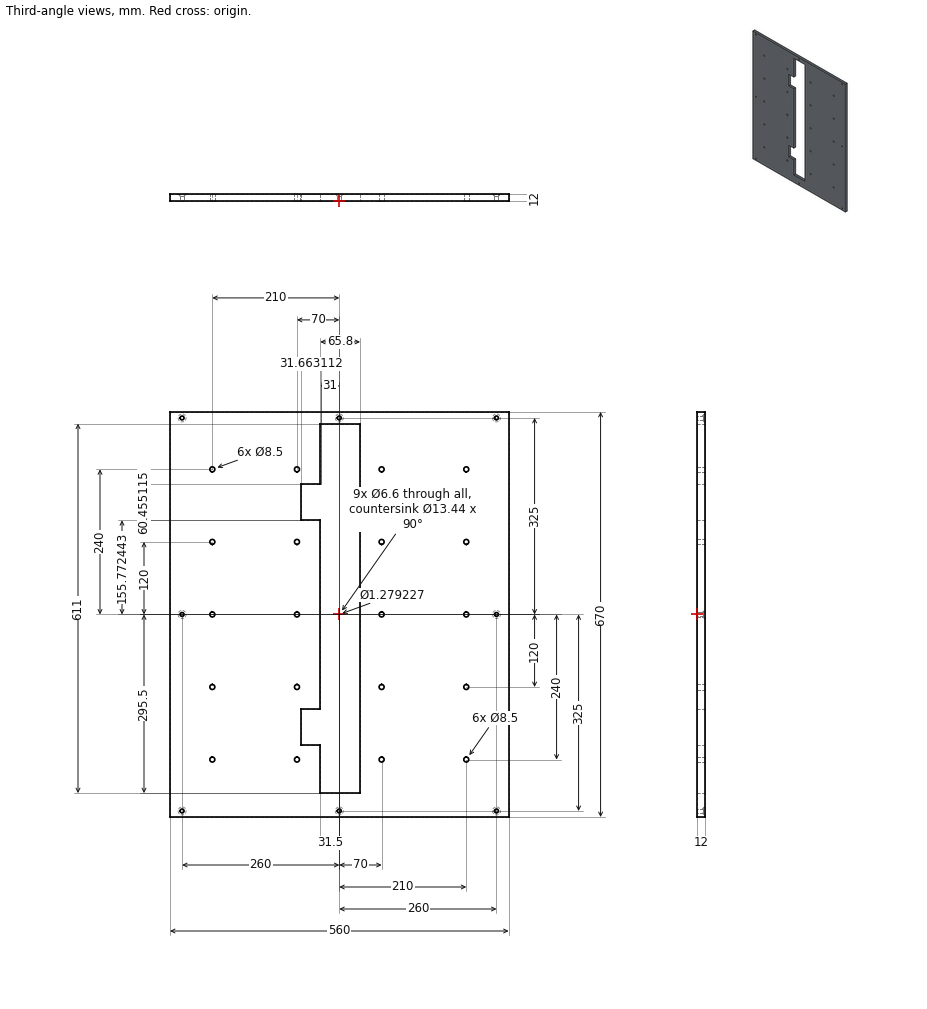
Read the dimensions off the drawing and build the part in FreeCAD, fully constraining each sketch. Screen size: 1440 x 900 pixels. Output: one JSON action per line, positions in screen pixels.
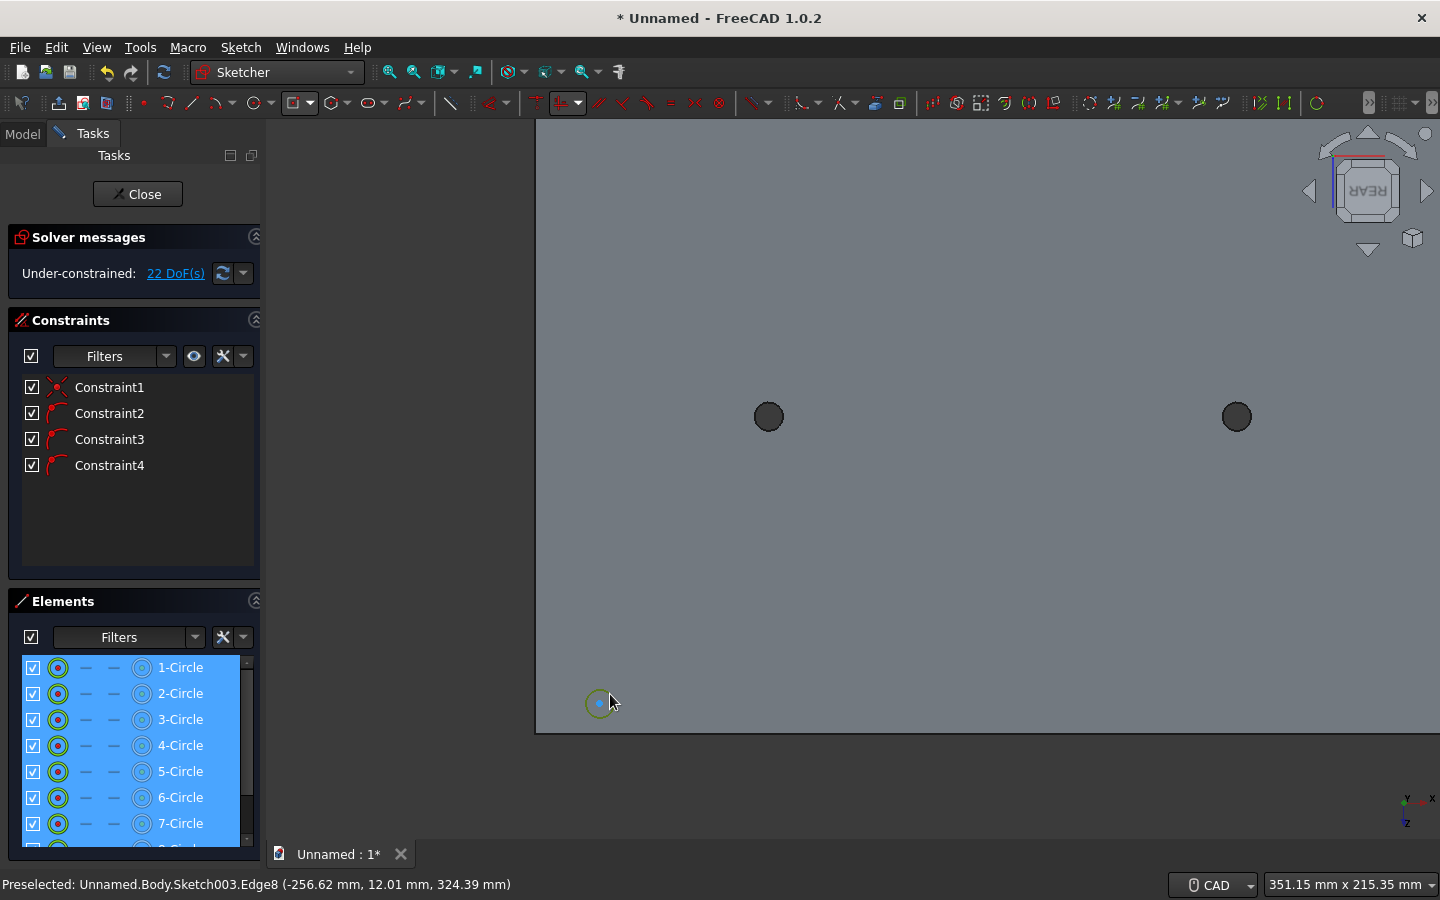
{"action": "scroll", "coordinate": [611, 698], "scroll_direction": "down", "scroll_amount": 8}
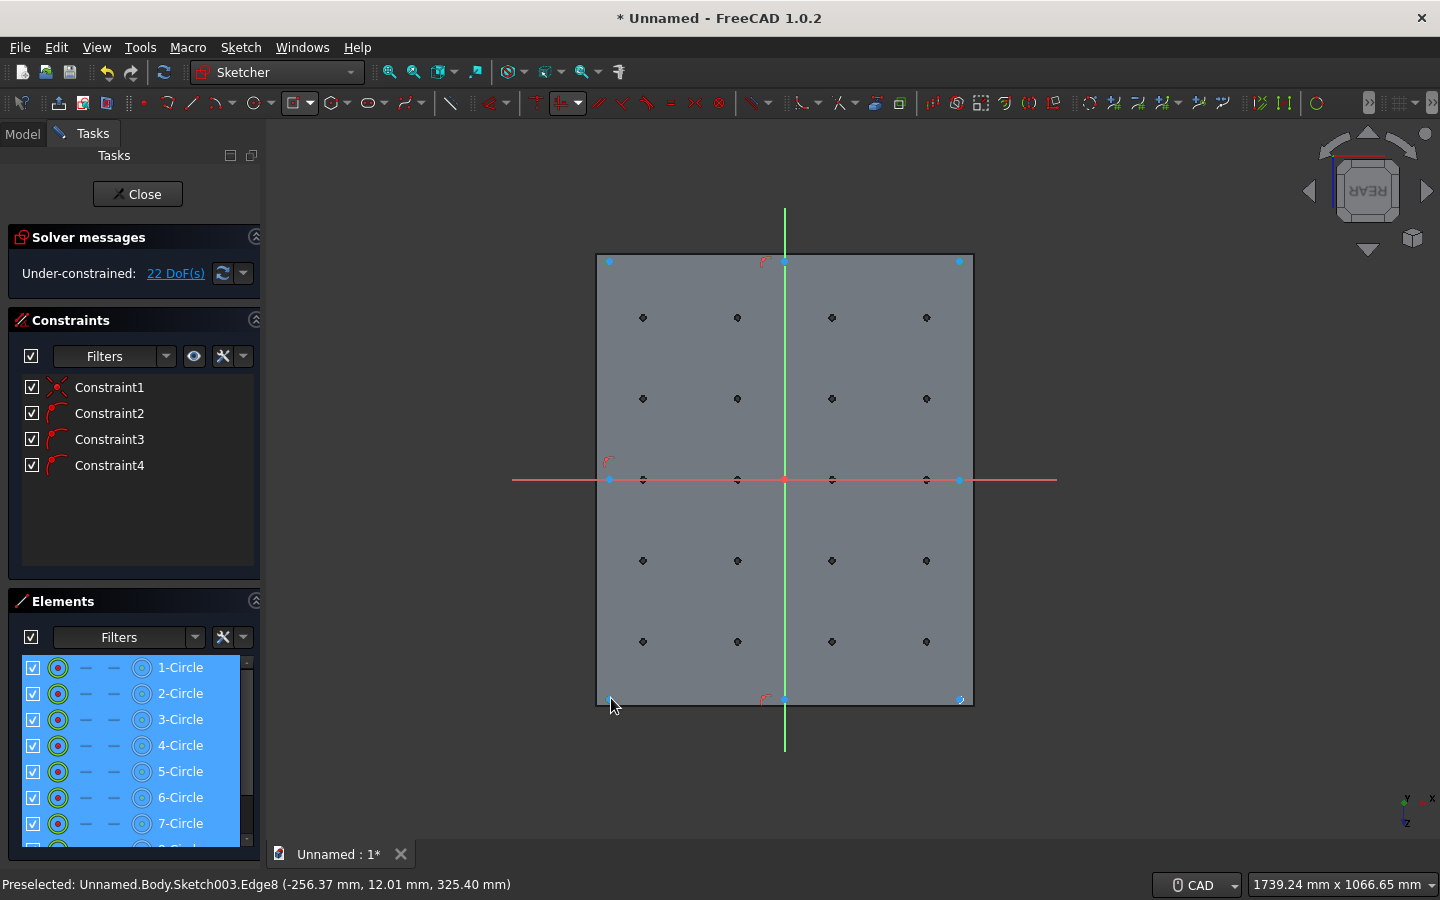
{"action": "scroll", "coordinate": [962, 698], "scroll_direction": "up", "scroll_amount": 8}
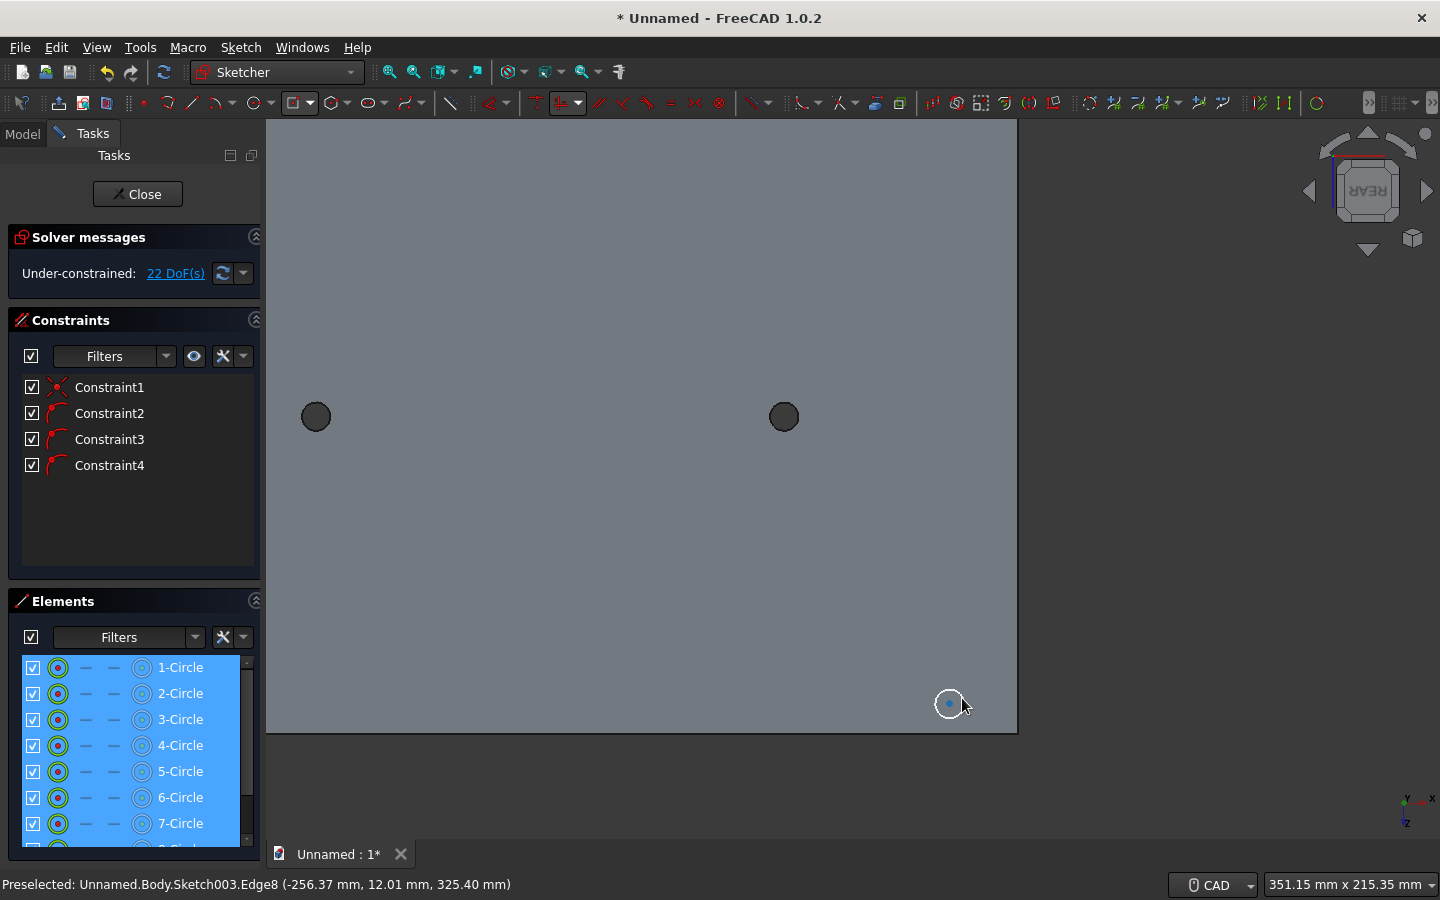
{"action": "left_click", "coordinate": [960, 694]}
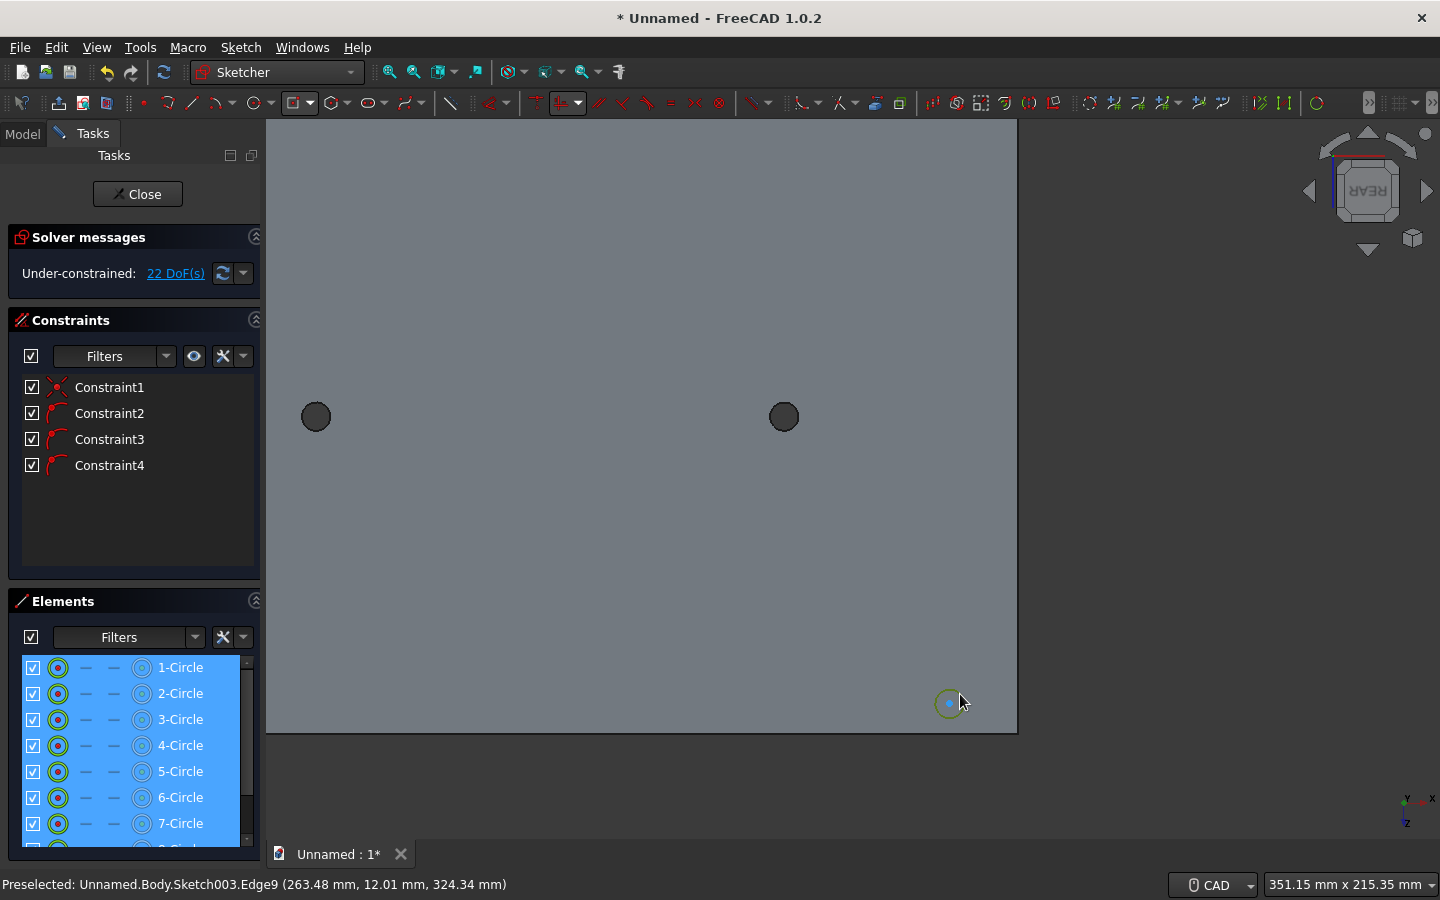
{"action": "left_click", "coordinate": [672, 104]}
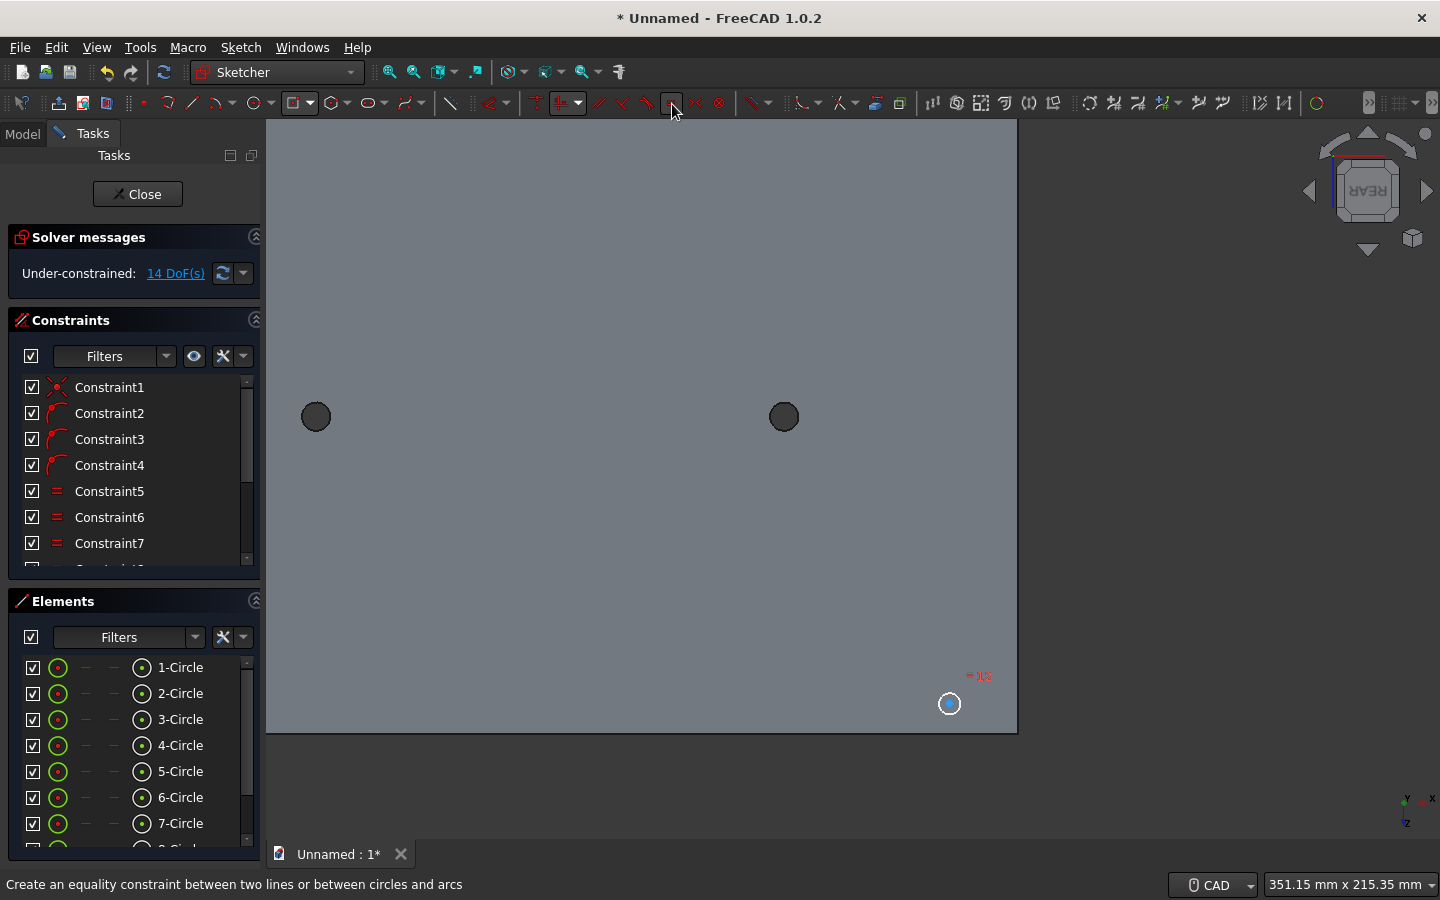
{"action": "scroll", "coordinate": [962, 698], "scroll_direction": "down", "scroll_amount": 8}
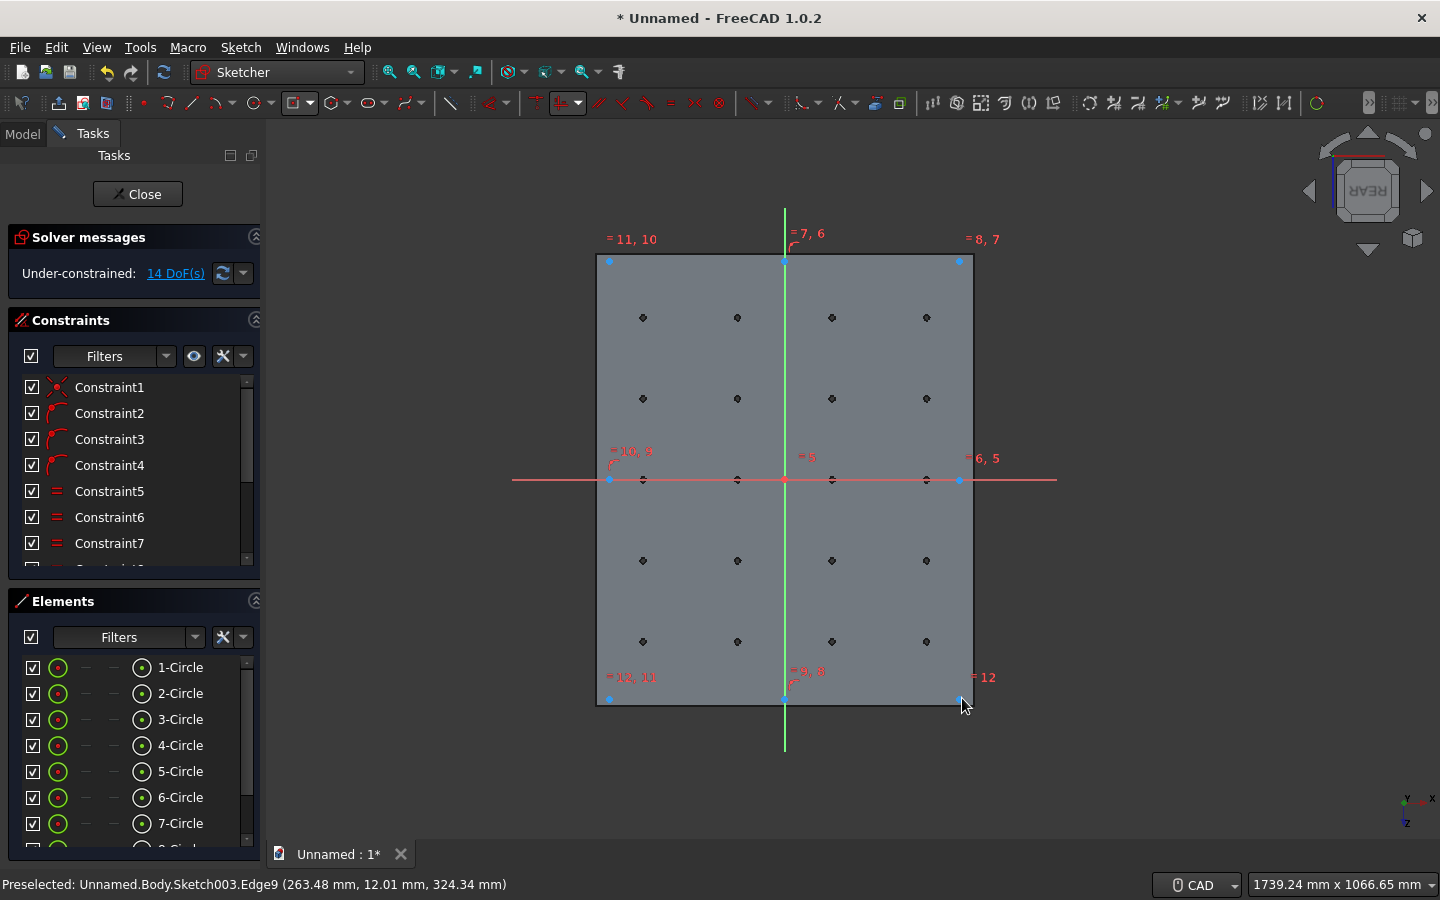
{"action": "left_click", "coordinate": [960, 481]}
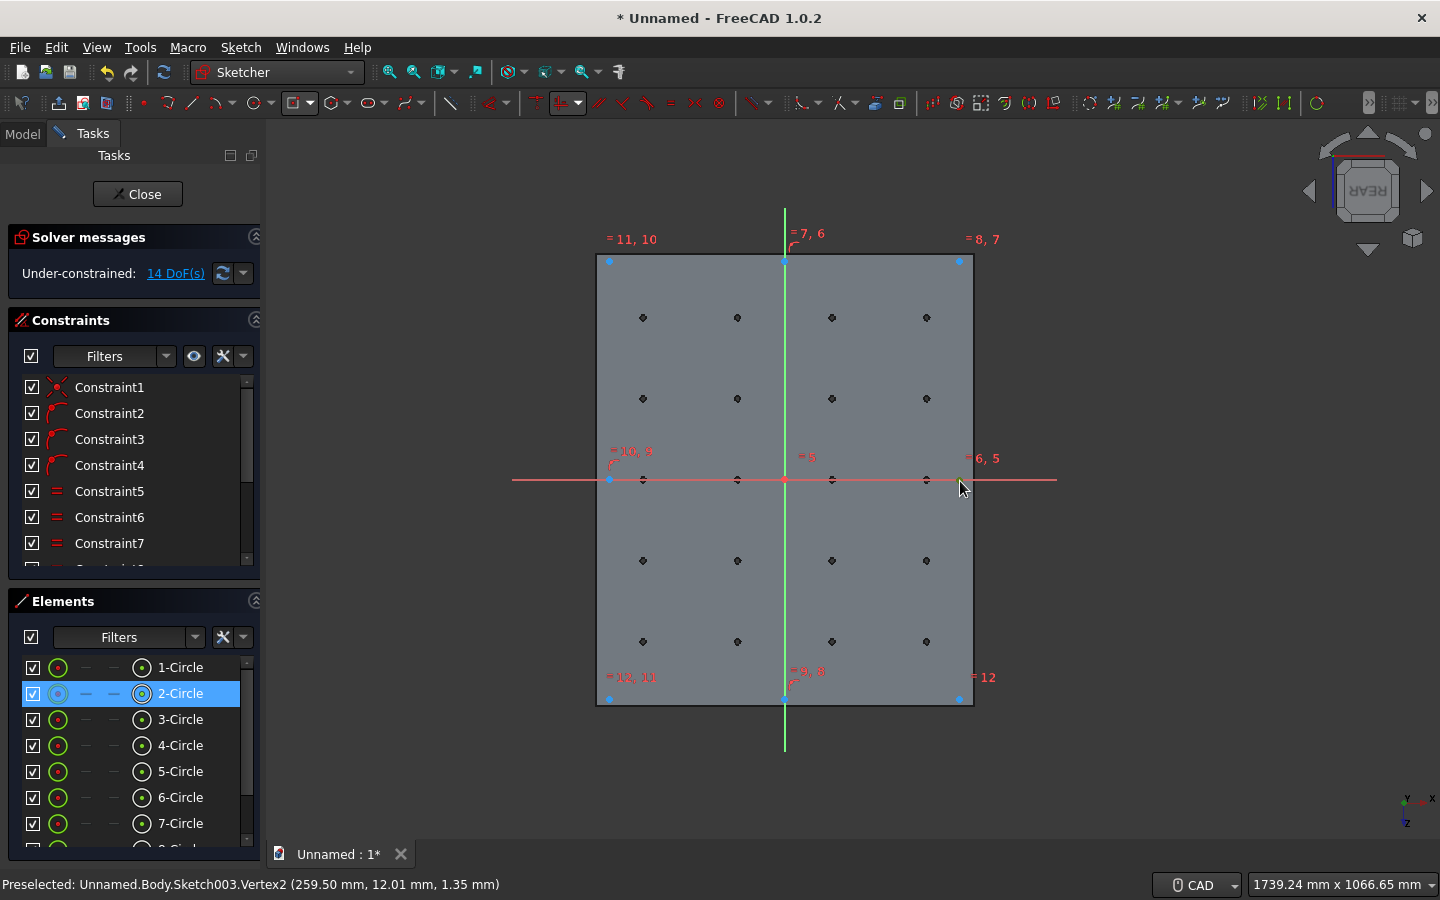
{"action": "left_click", "coordinate": [574, 480]}